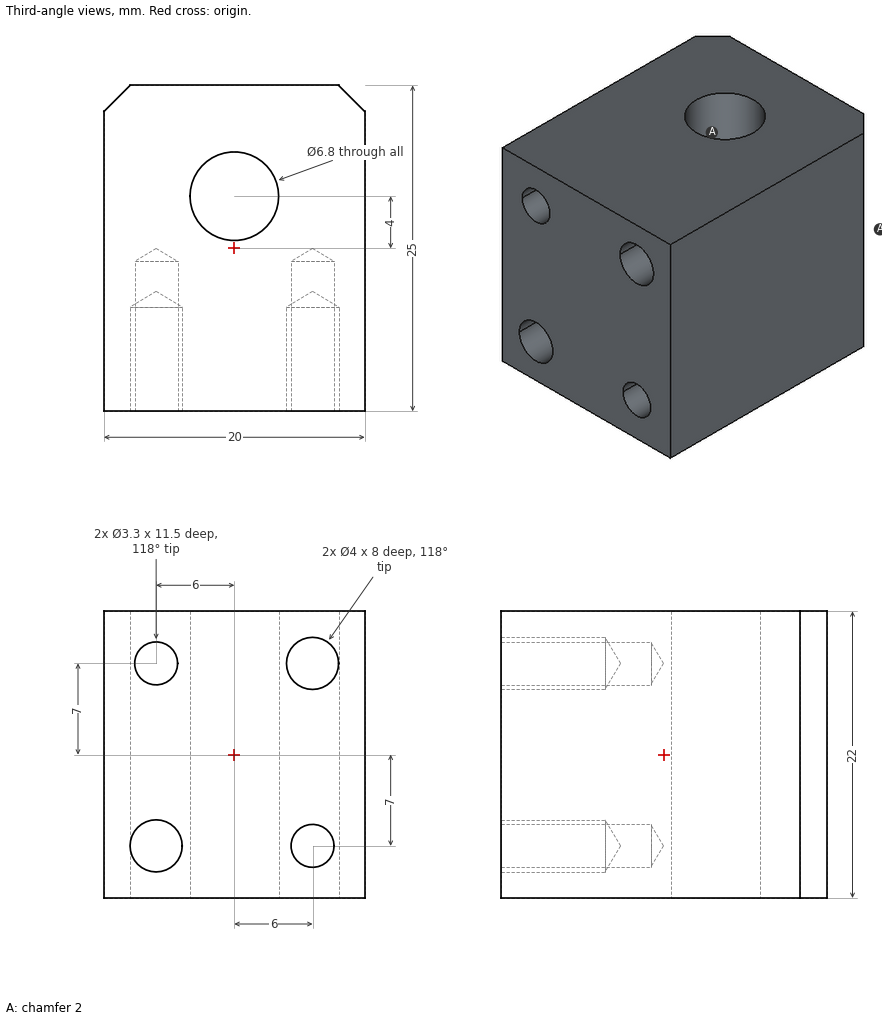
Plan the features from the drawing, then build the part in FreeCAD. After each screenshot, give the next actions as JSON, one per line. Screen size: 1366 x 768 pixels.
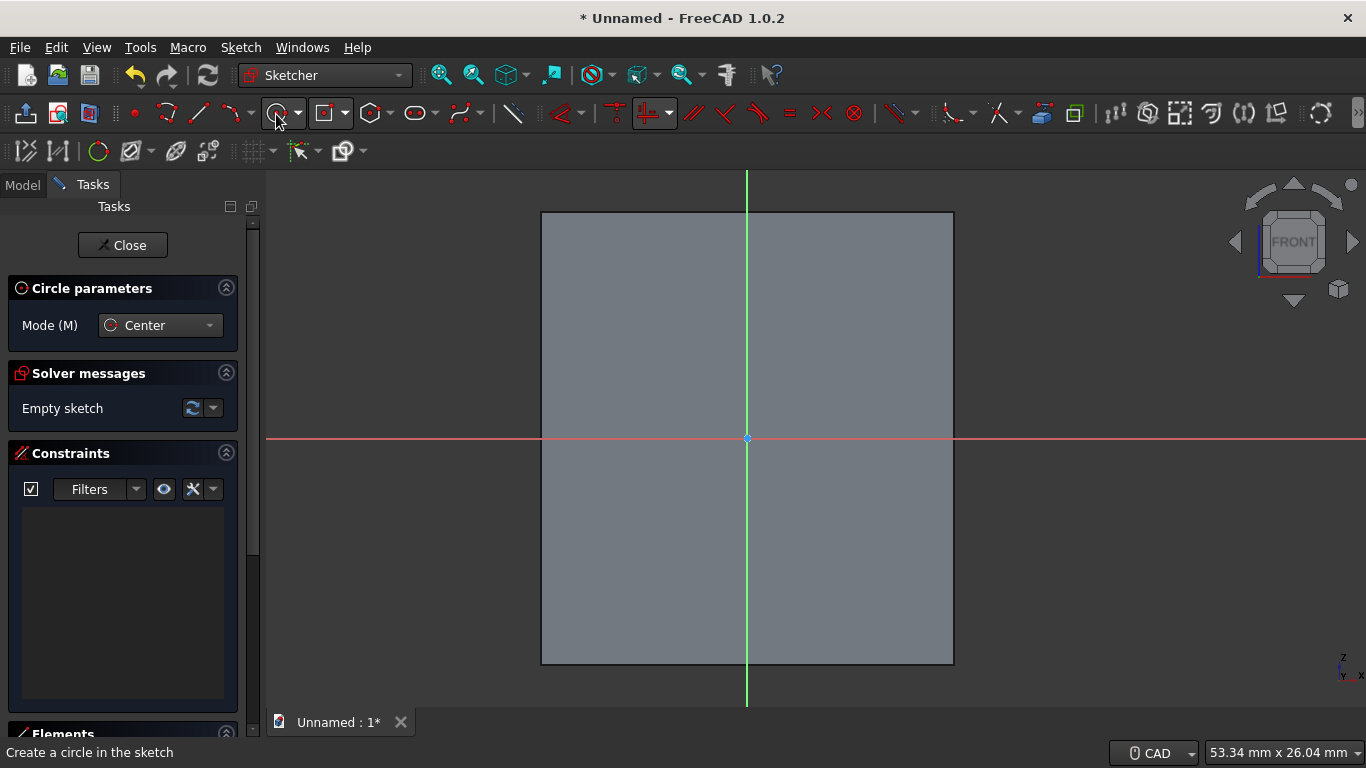
{"action": "left_click", "coordinate": [624, 294]}
{"action": "mouse_move", "coordinate": [648, 270]}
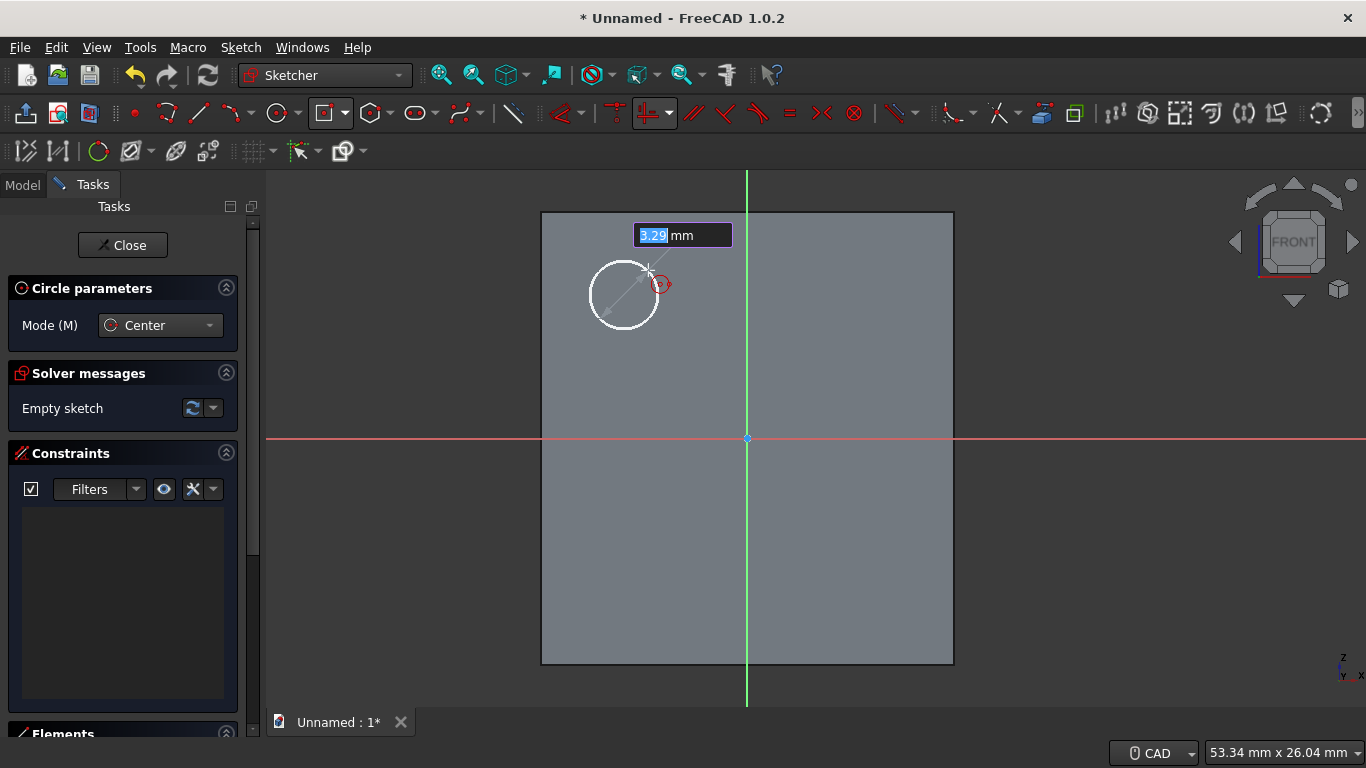
{"action": "type", "text": "3.3"}
{"action": "key", "text": "Return"}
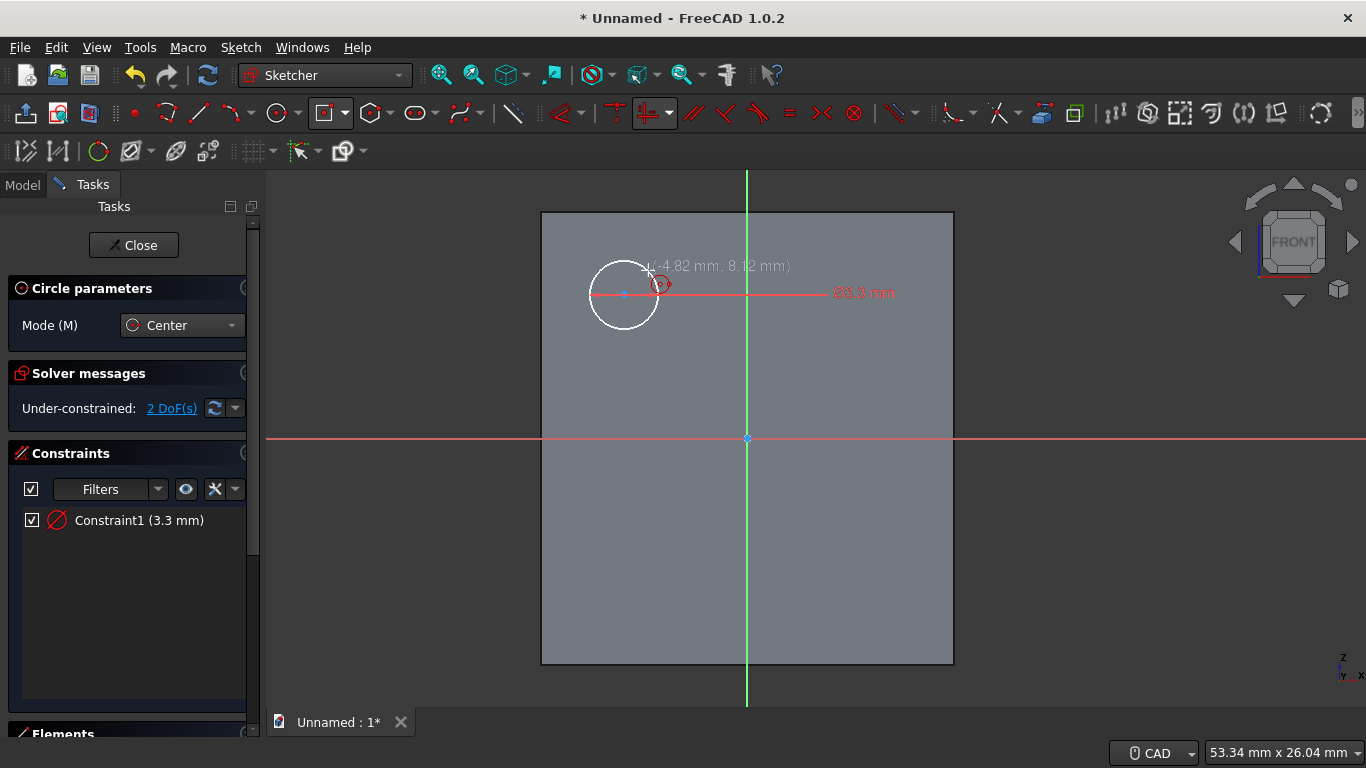
{"action": "left_click", "coordinate": [871, 583]}
{"action": "mouse_move", "coordinate": [895, 559]}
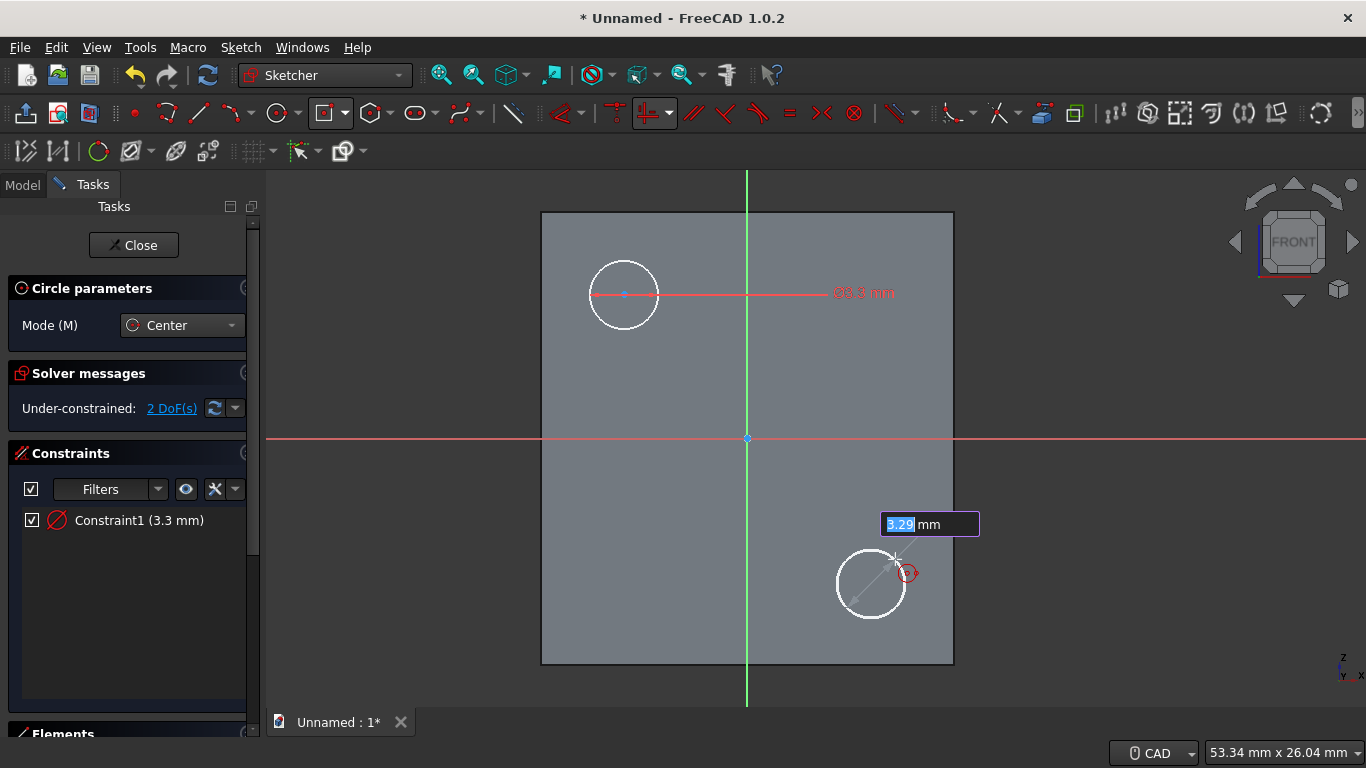
{"action": "type", "text": "3.3"}
{"action": "key", "text": "Return"}
{"action": "key", "text": "Escape"}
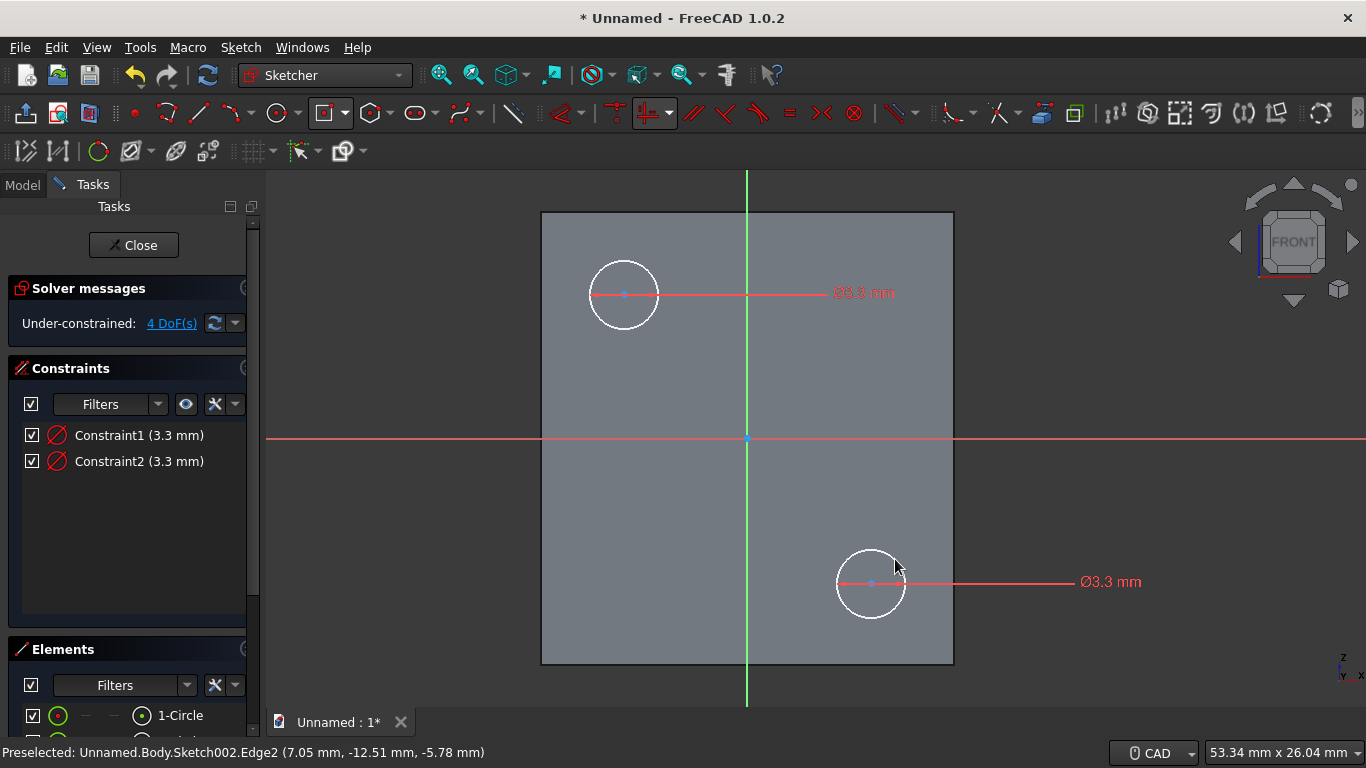
{"action": "left_click", "coordinate": [624, 295]}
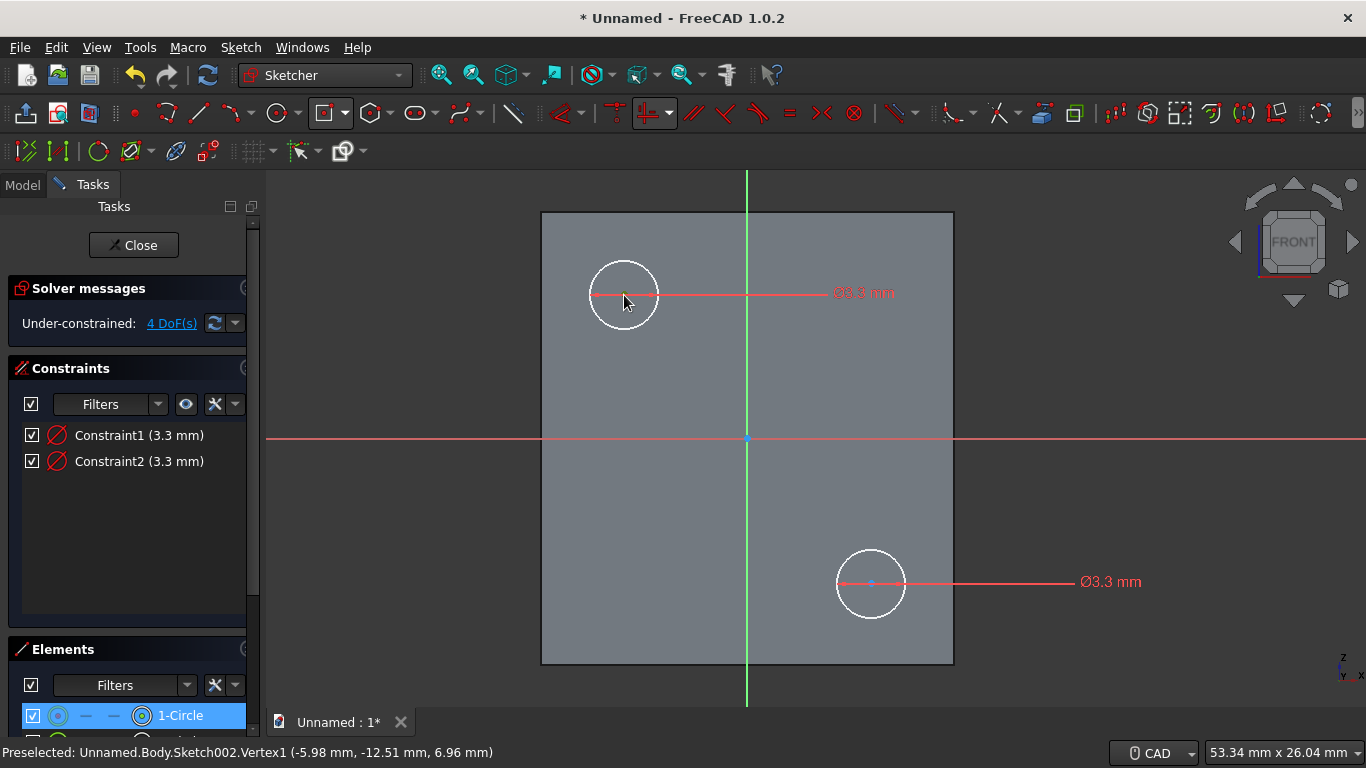
{"action": "key", "text": "l"}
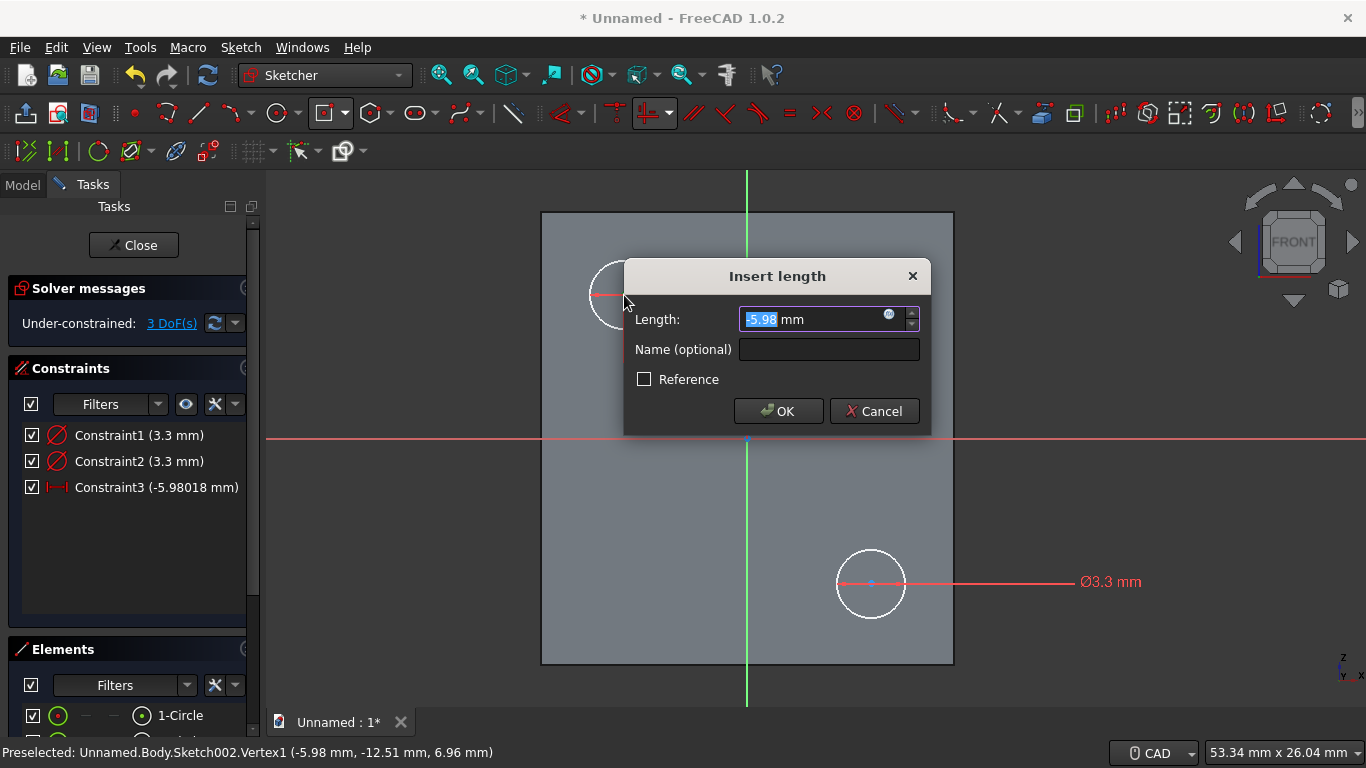
{"action": "type", "text": "-6"}
{"action": "key", "text": "Return"}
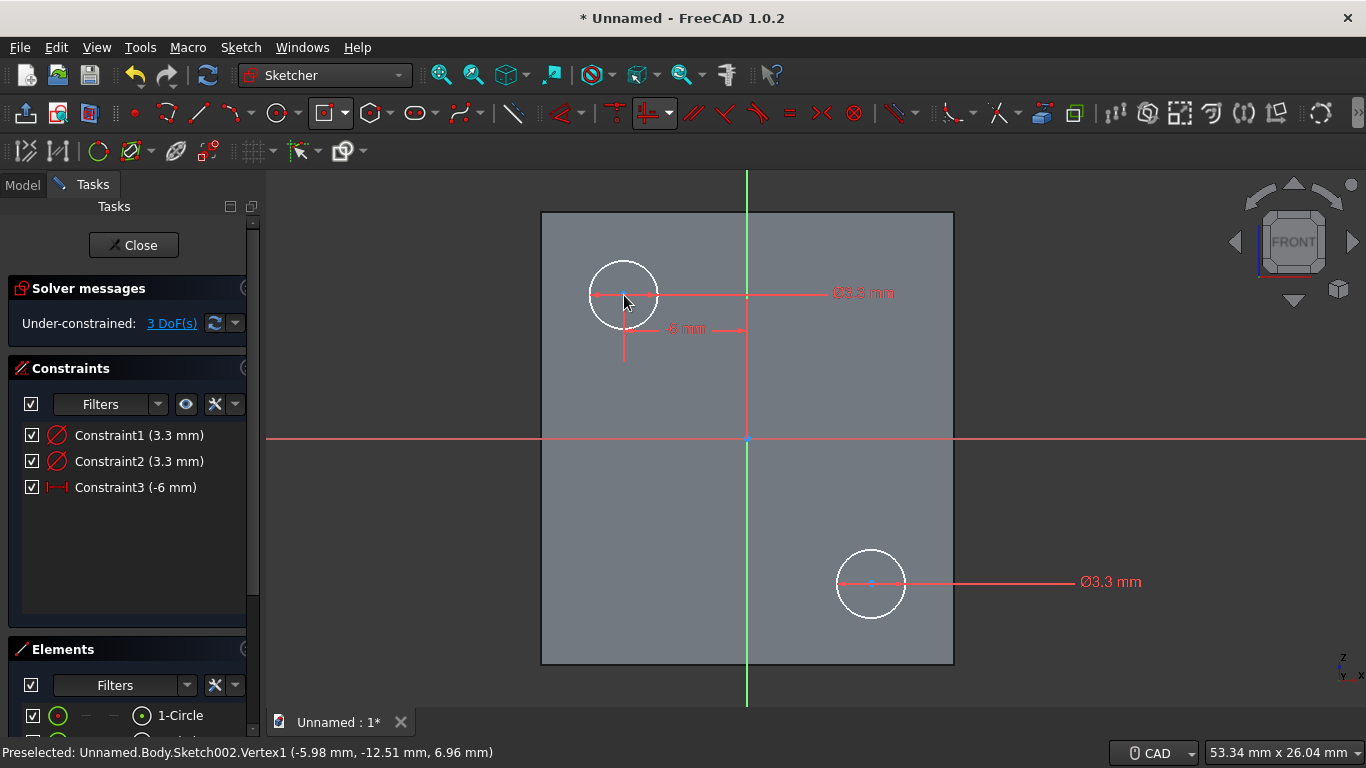
{"action": "left_click", "coordinate": [624, 295]}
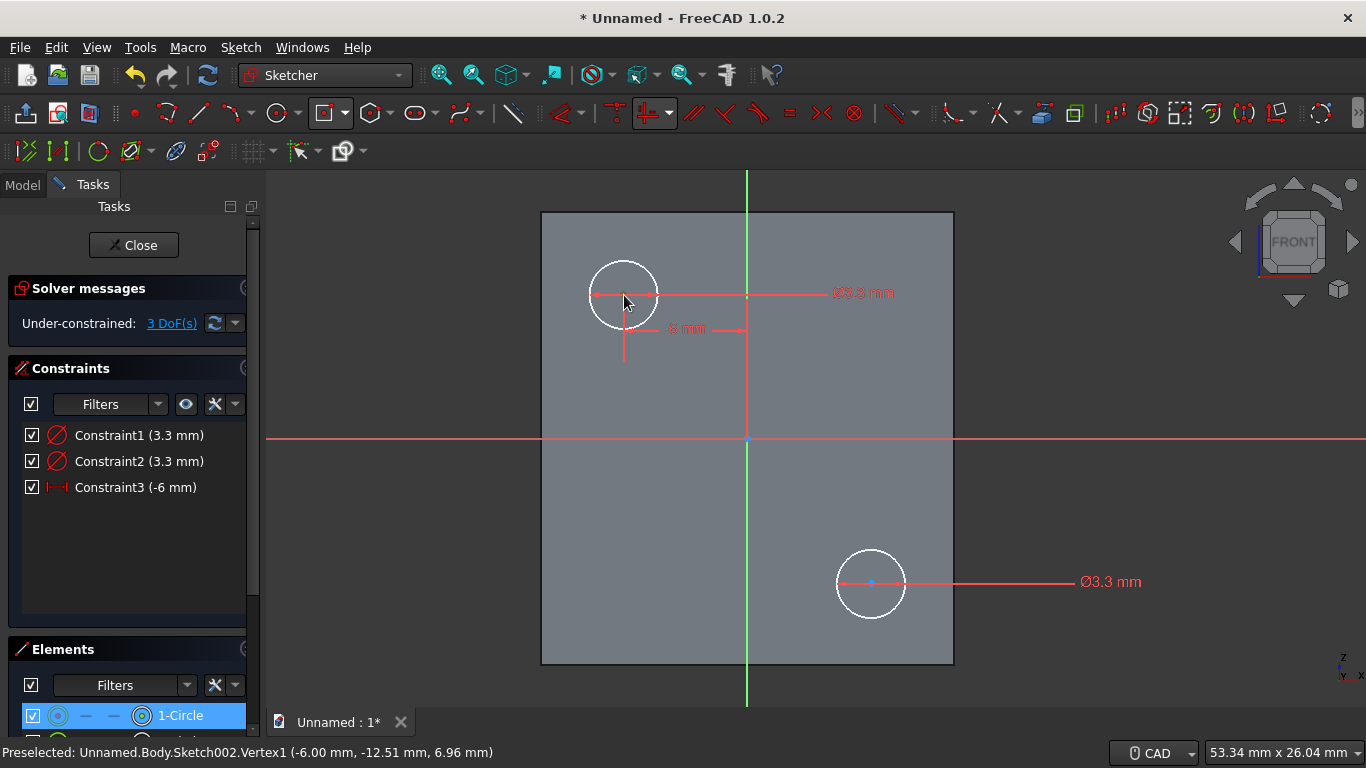
{"action": "left_click", "coordinate": [584, 114]}